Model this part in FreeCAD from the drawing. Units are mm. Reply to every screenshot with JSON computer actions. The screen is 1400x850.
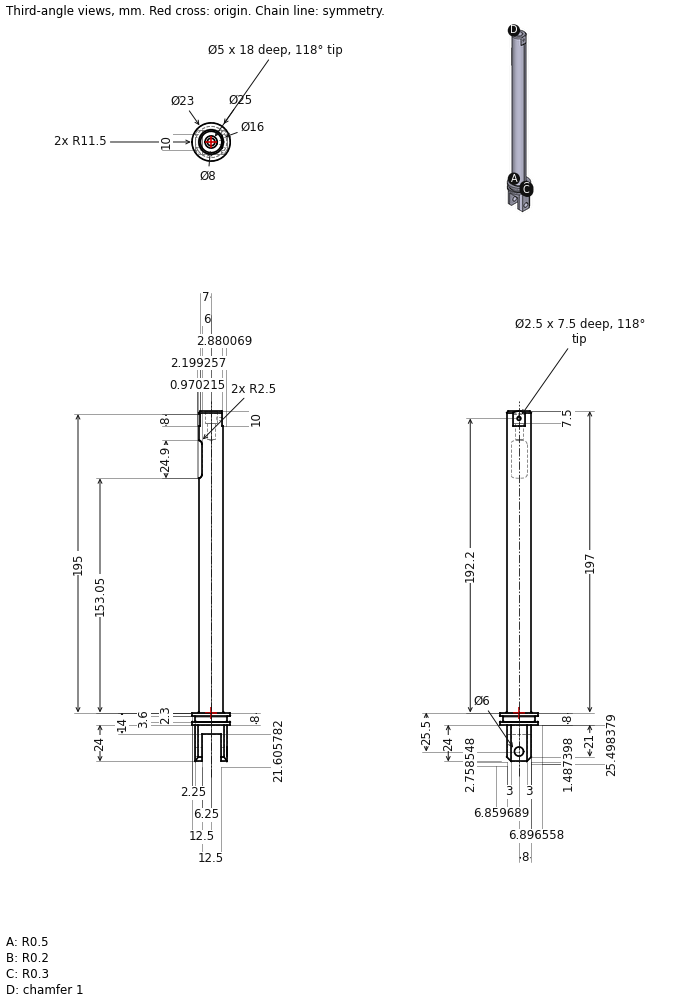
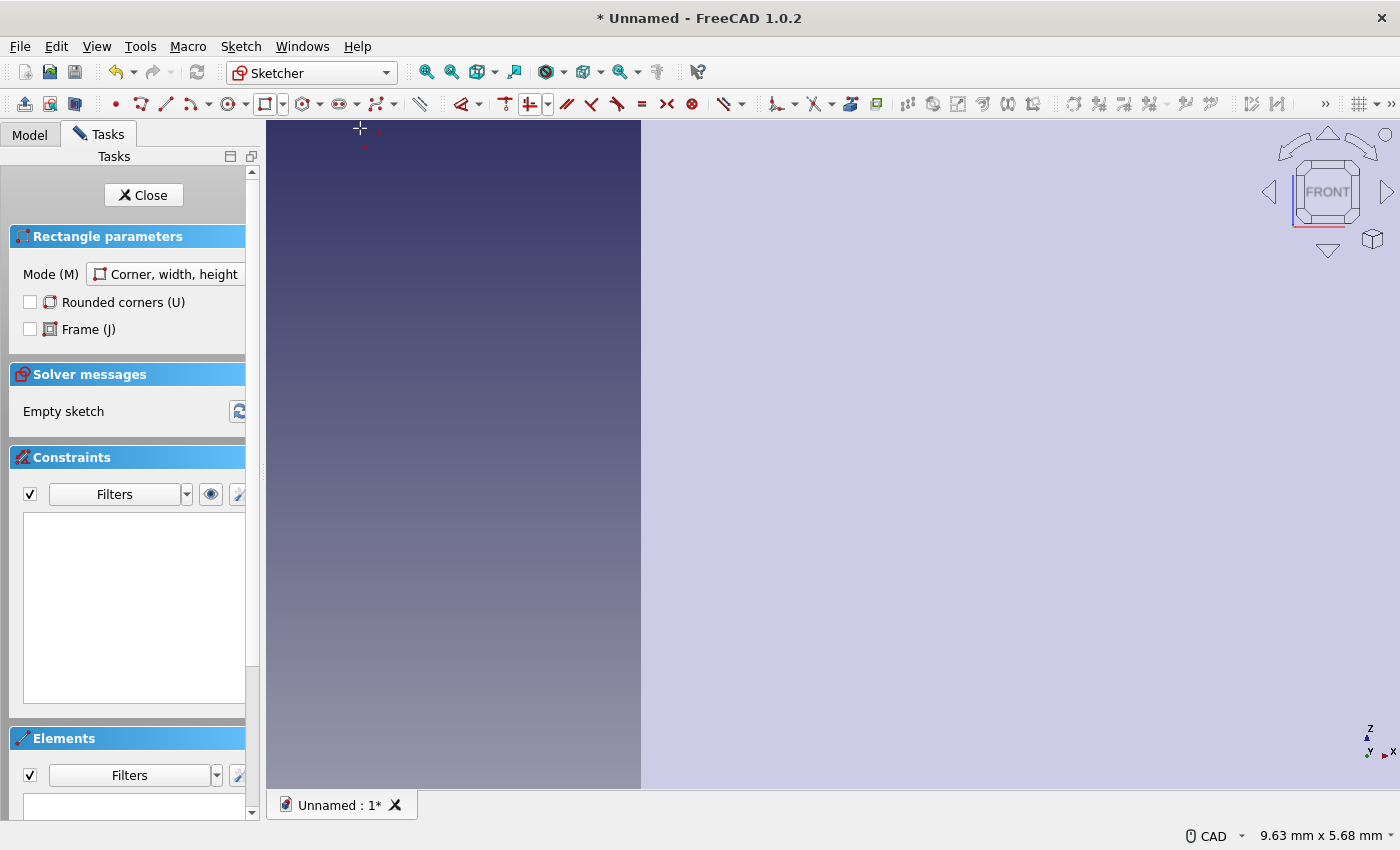
{"action": "left_click", "coordinate": [631, 239]}
{"action": "mouse_move", "coordinate": [895, 663]}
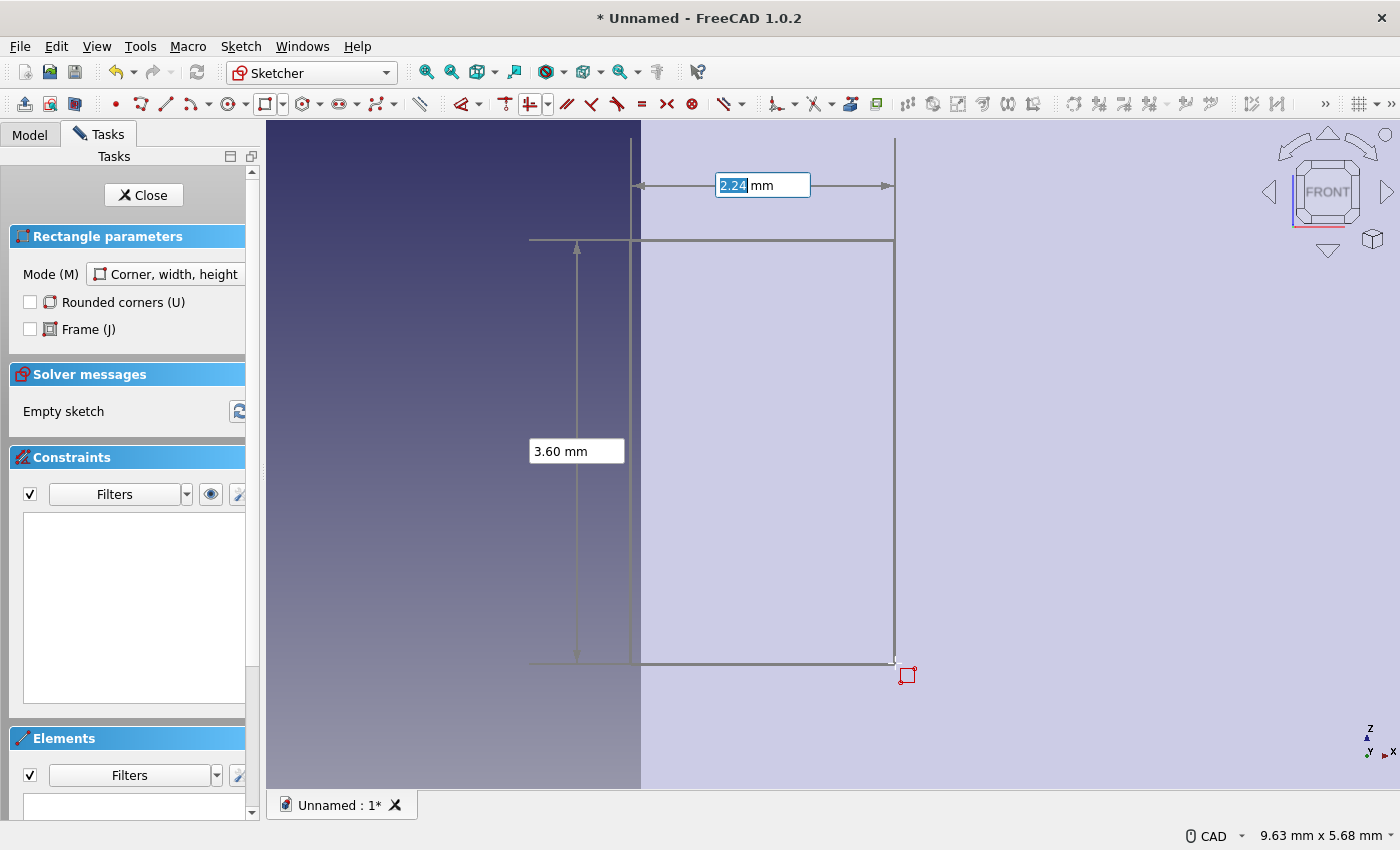
{"action": "type", "text": "2.25"}
{"action": "key", "text": "Tab"}
{"action": "type", "text": "3.6"}
{"action": "key", "text": "Return"}
{"action": "key", "text": "Escape"}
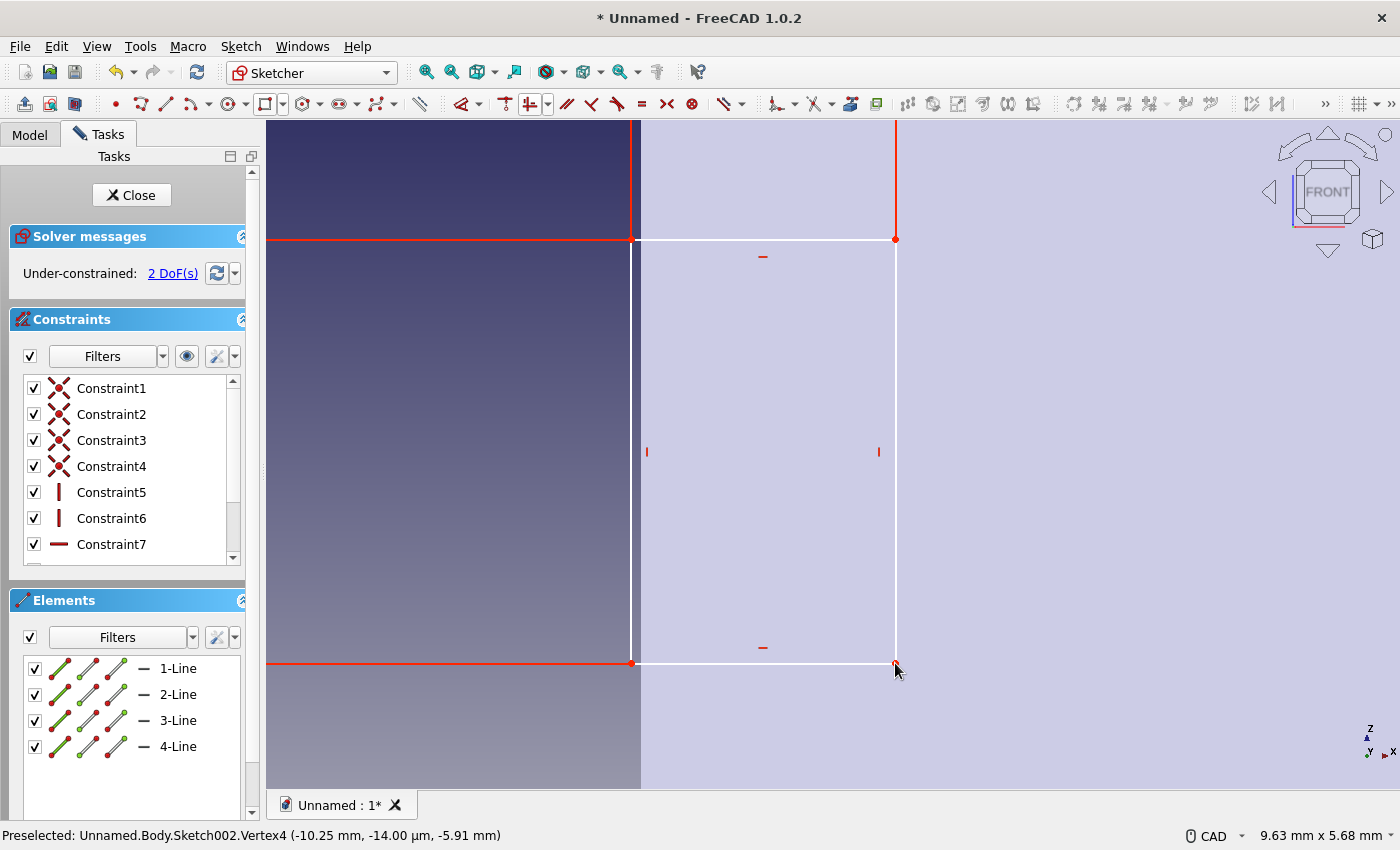
{"action": "left_click", "coordinate": [460, 104]}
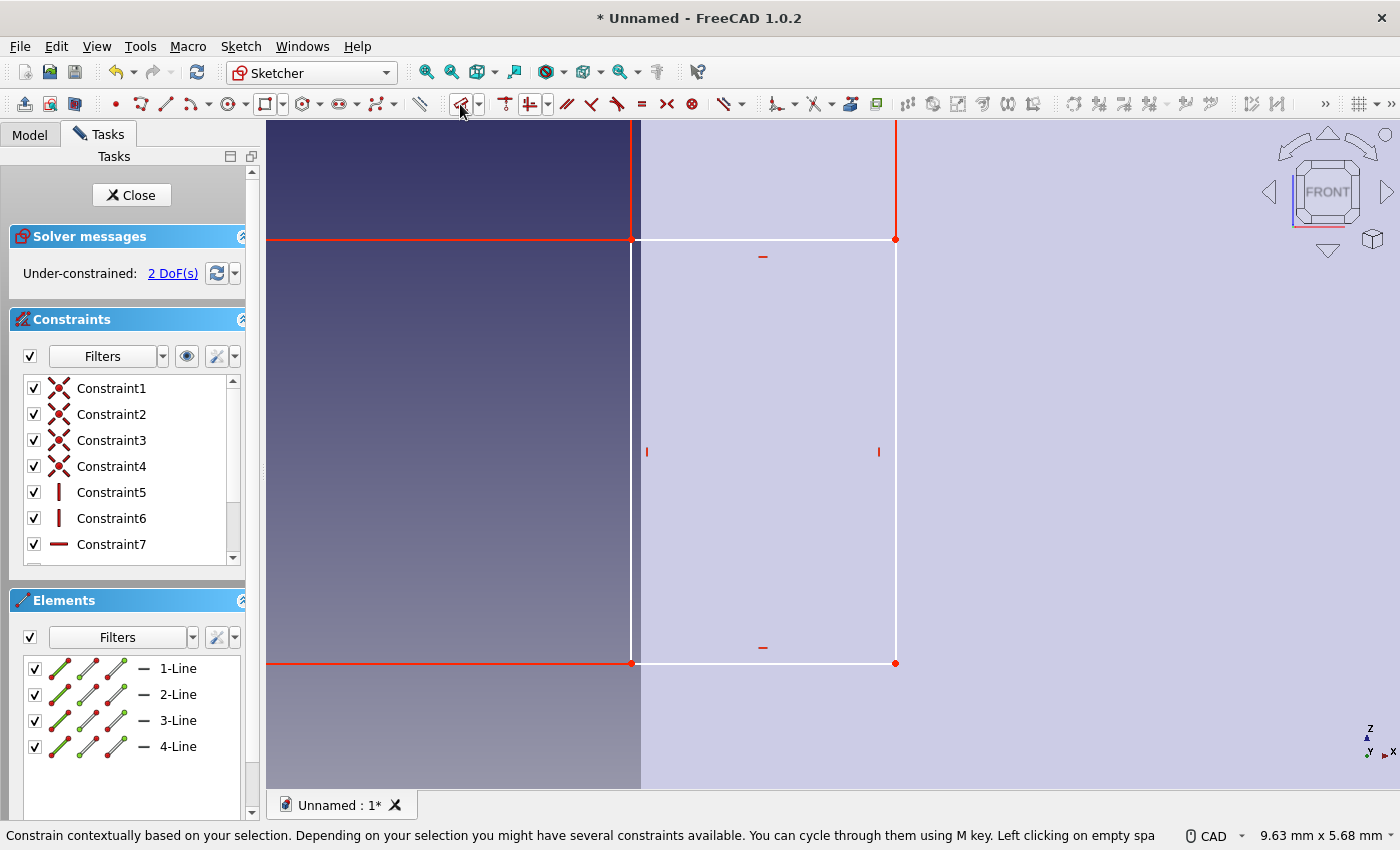
{"action": "left_click", "coordinate": [631, 240]}
{"action": "left_click", "coordinate": [597, 194]}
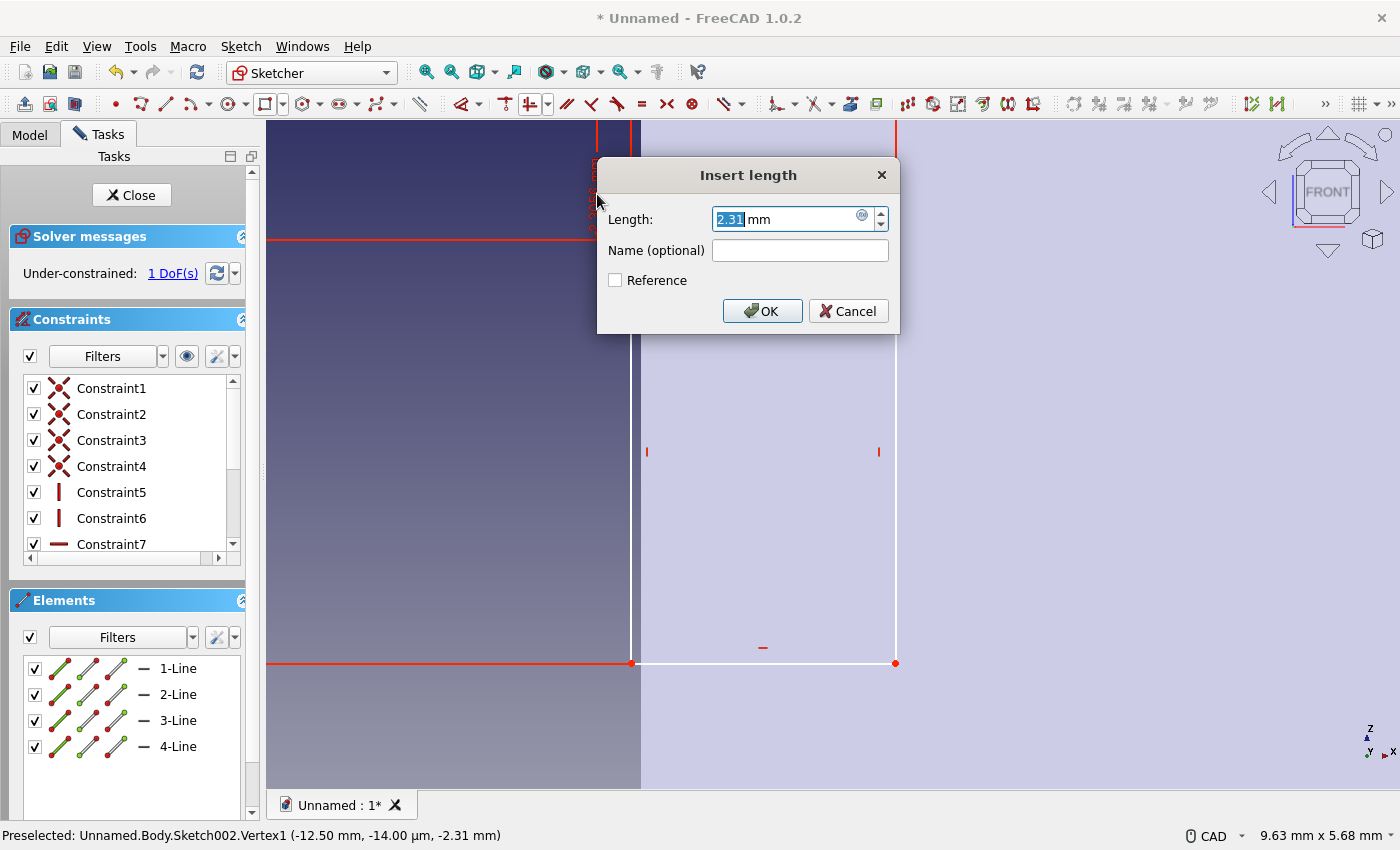
{"action": "type", "text": "2.3"}
{"action": "key", "text": "Return"}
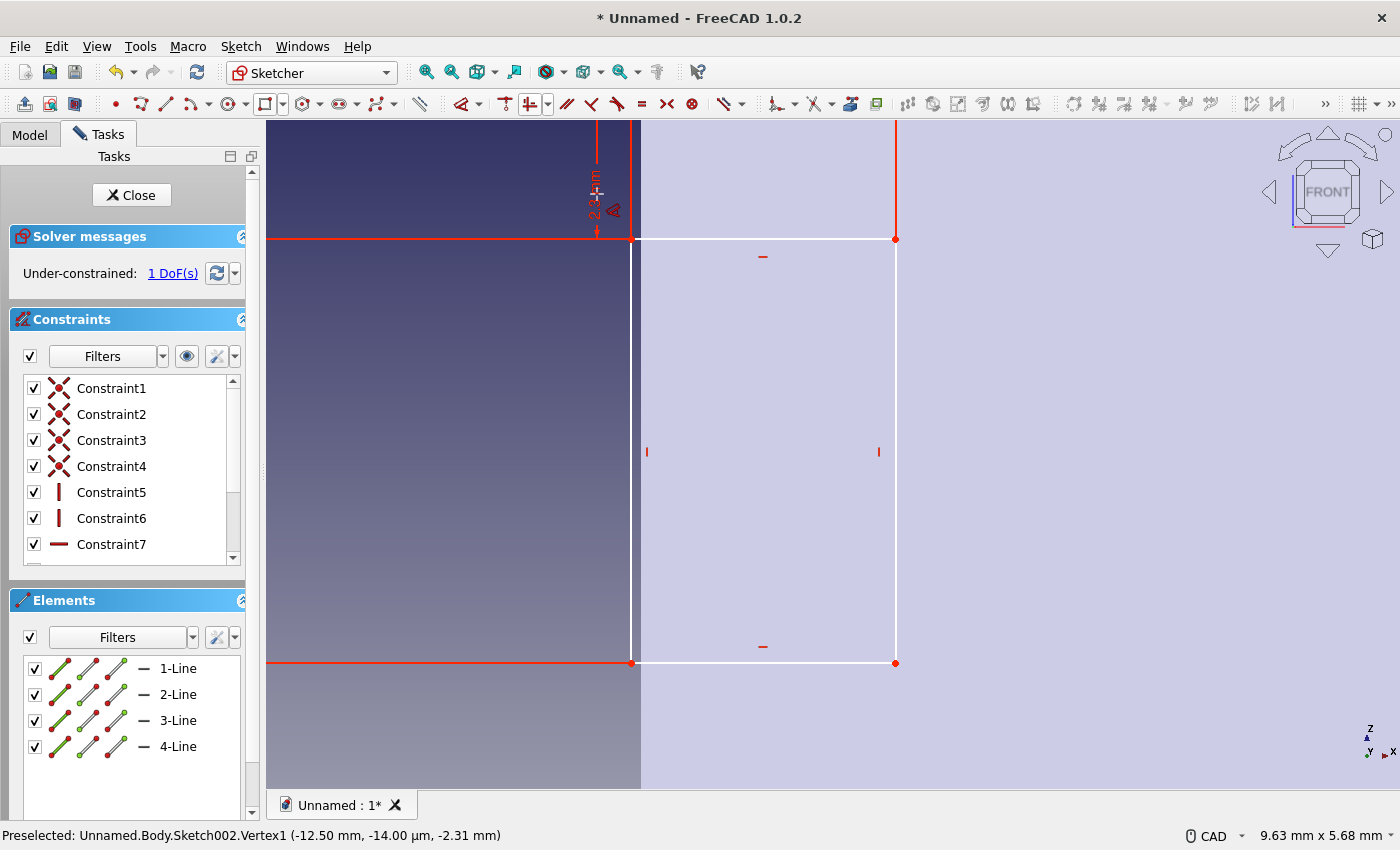
{"action": "left_click", "coordinate": [631, 239]}
{"action": "left_click", "coordinate": [933, 273]}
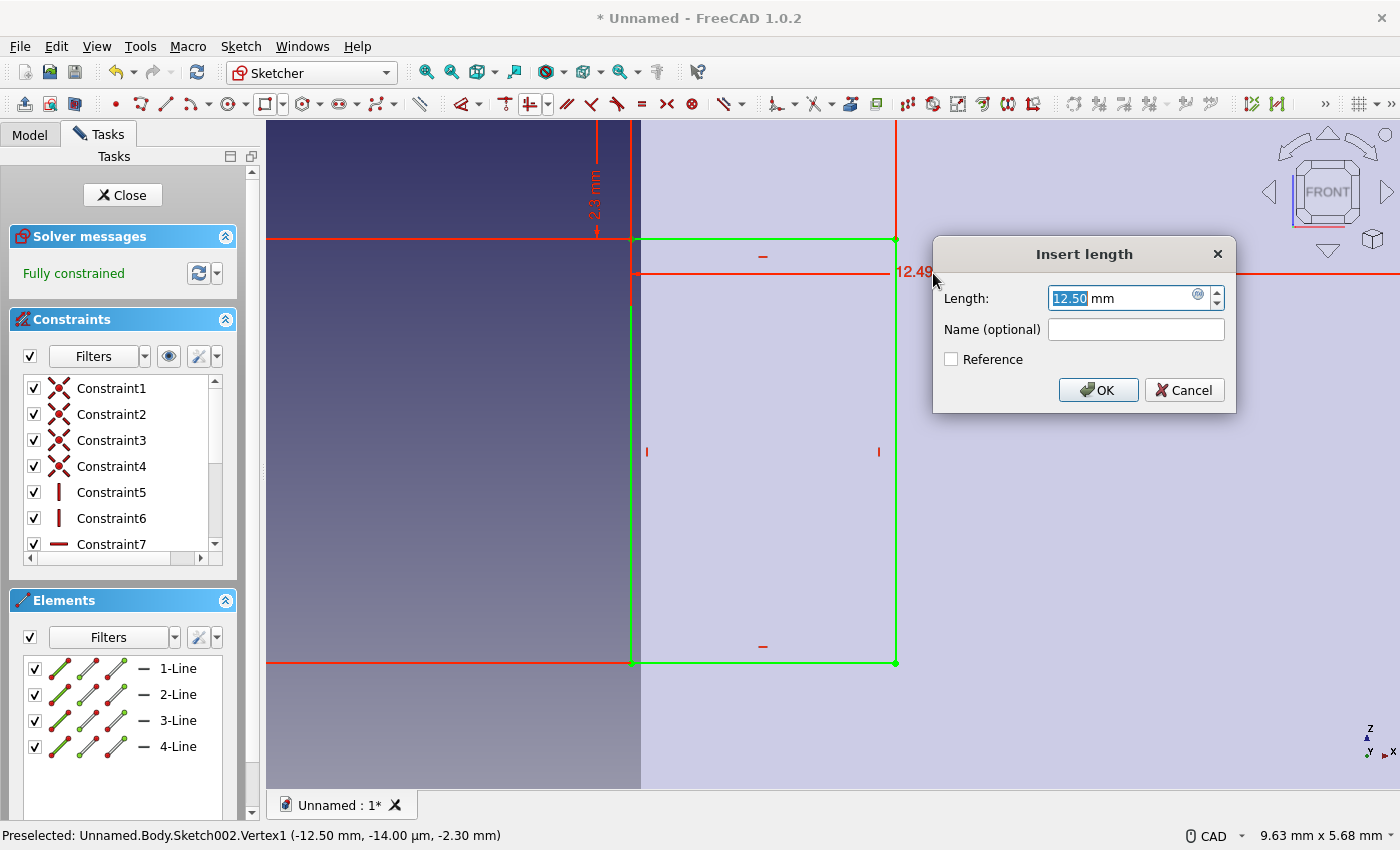
{"action": "type", "text": "12.5"}
{"action": "key", "text": "Return"}
{"action": "key", "text": "Escape"}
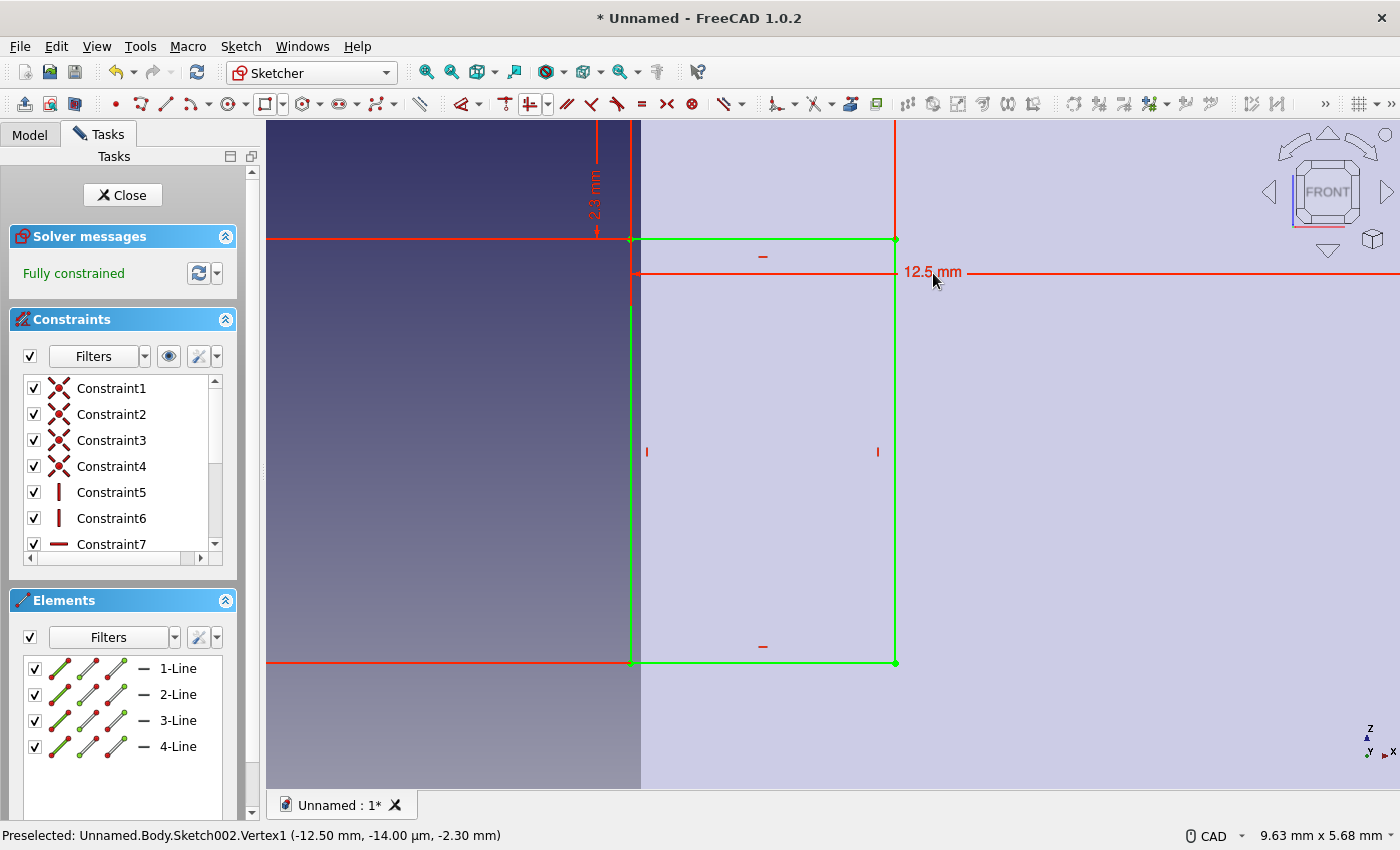
{"action": "left_click", "coordinate": [123, 195]}